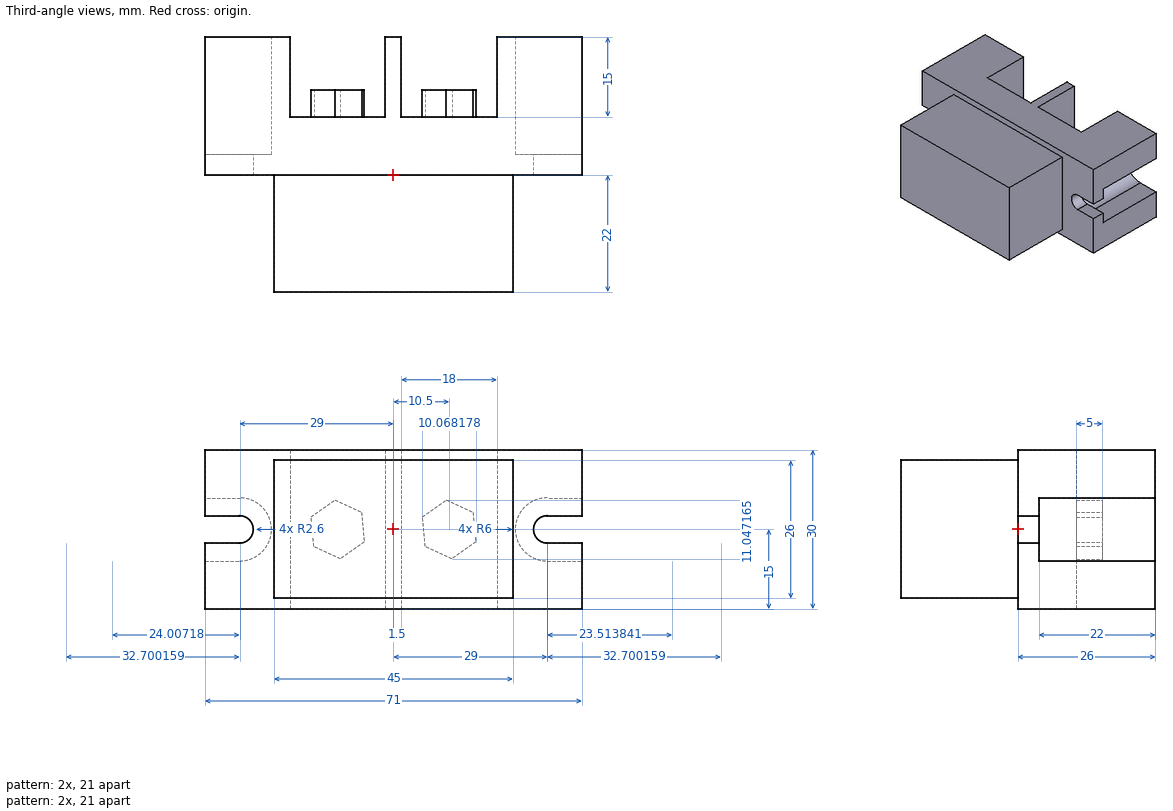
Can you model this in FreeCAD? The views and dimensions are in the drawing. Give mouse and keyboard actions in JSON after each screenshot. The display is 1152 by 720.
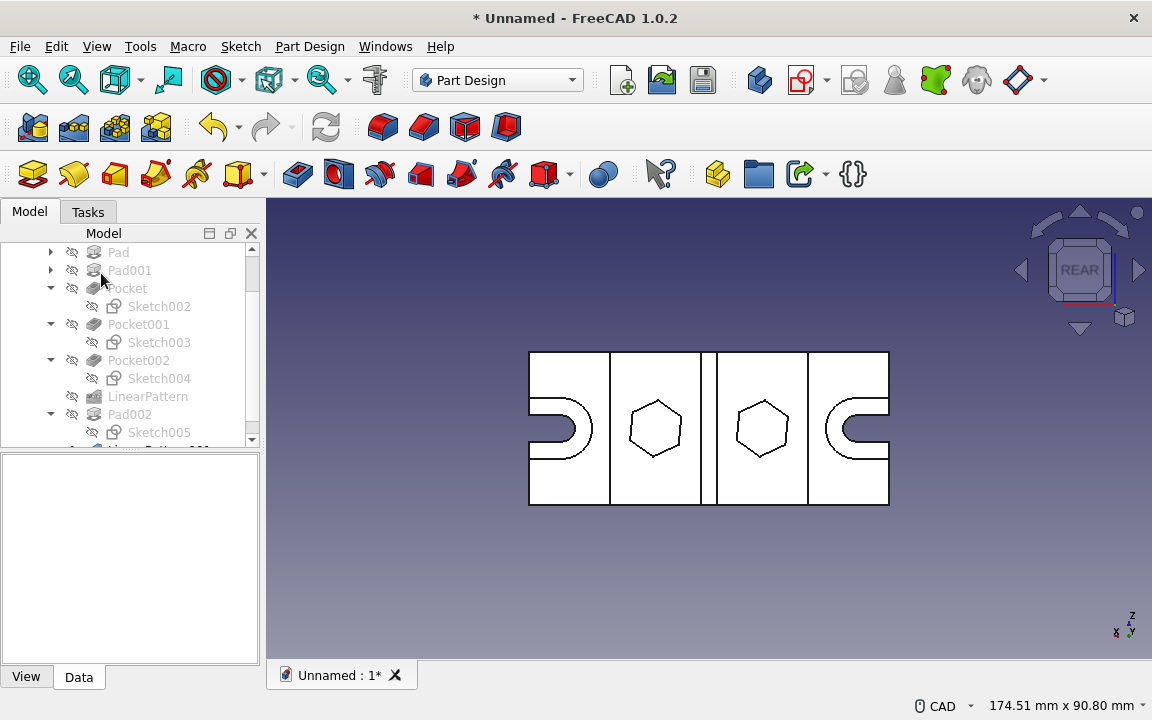
{"action": "key", "text": "0"}